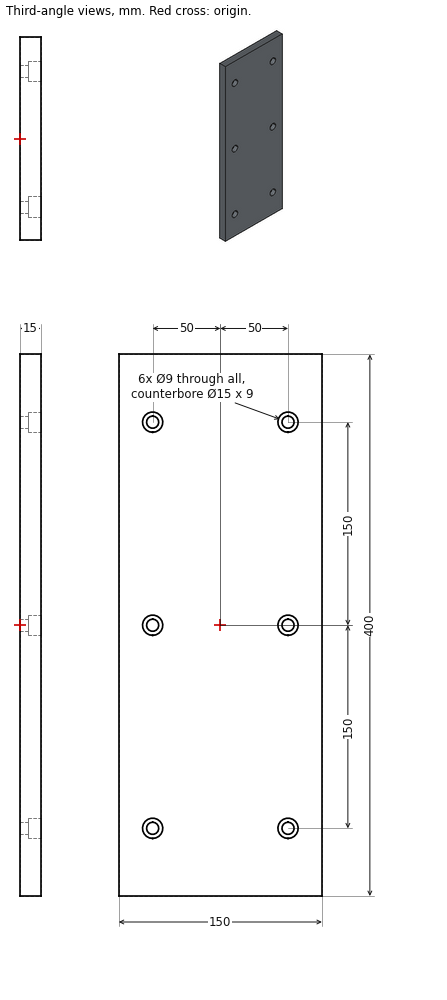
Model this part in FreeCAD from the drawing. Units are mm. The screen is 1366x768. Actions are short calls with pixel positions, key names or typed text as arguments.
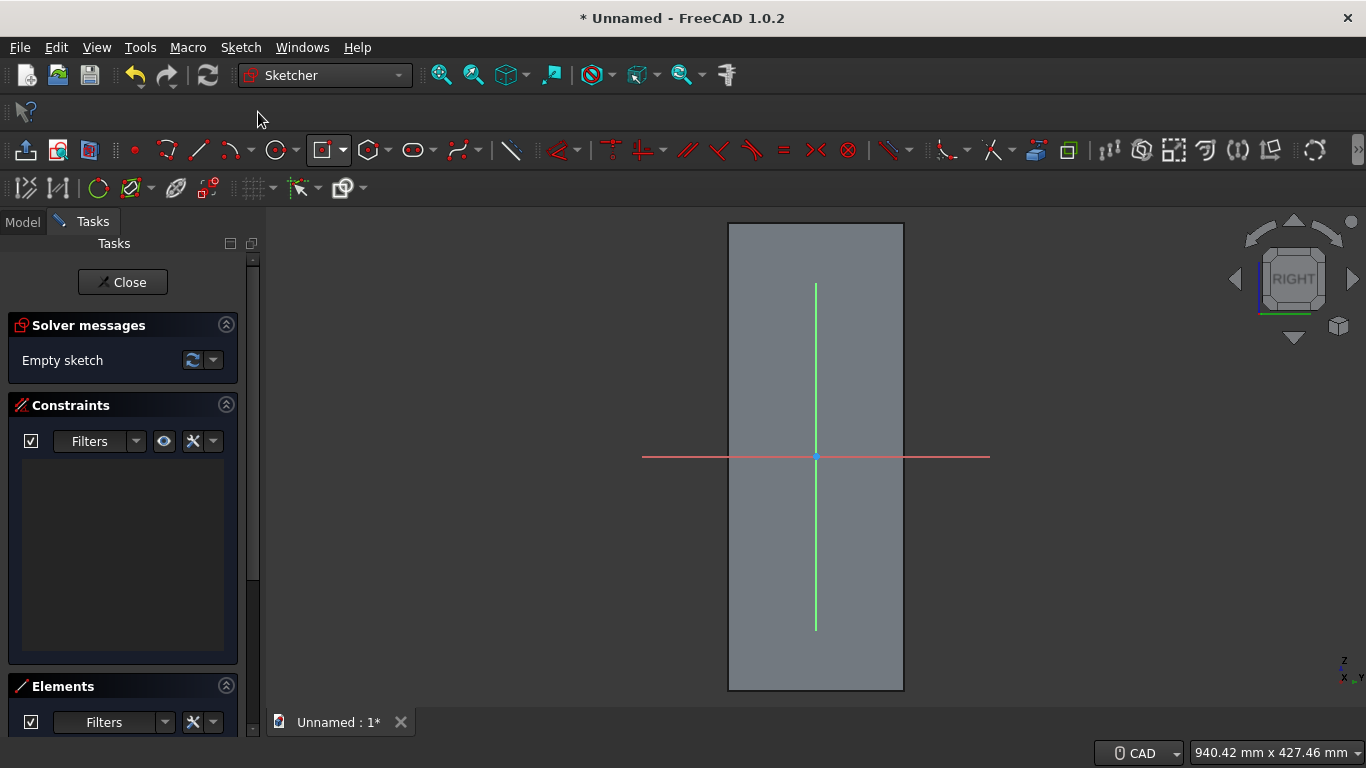
click(276, 150)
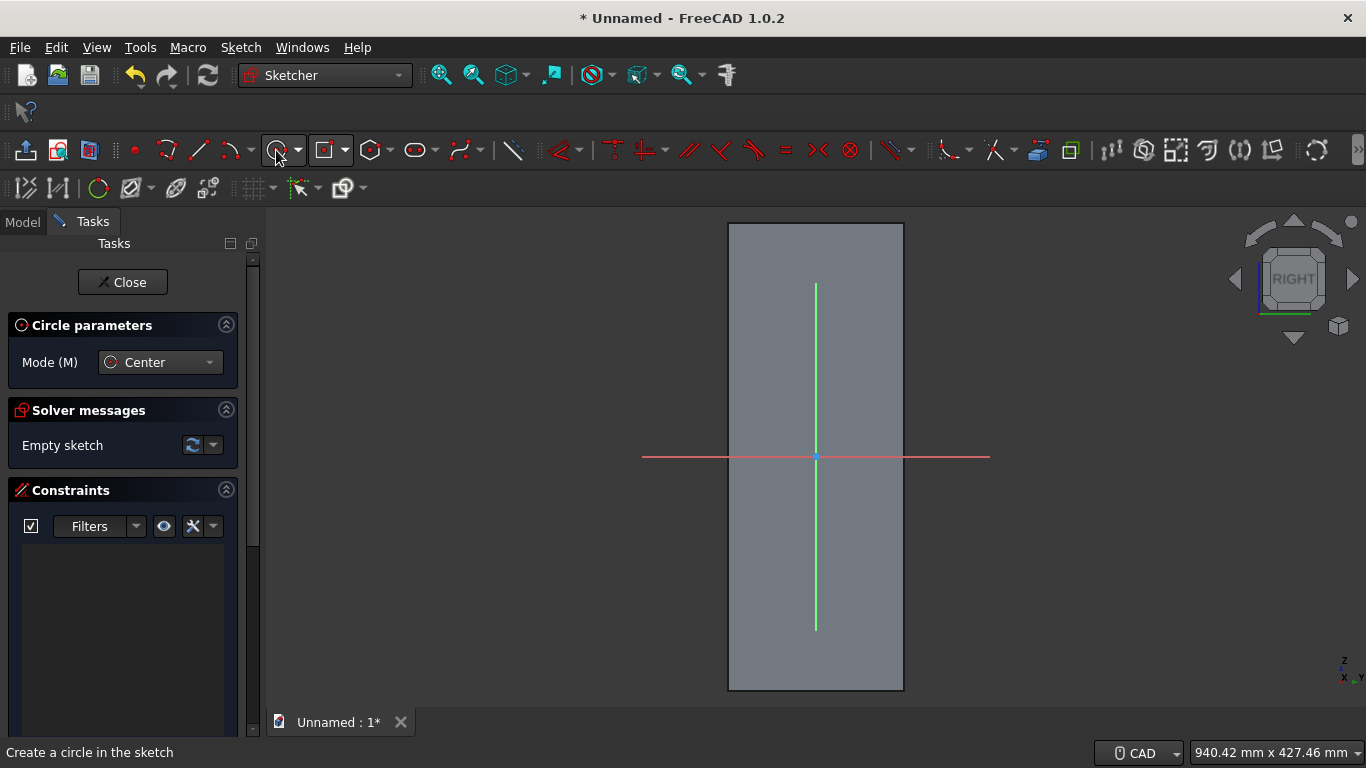
scroll(874, 282, up, 8)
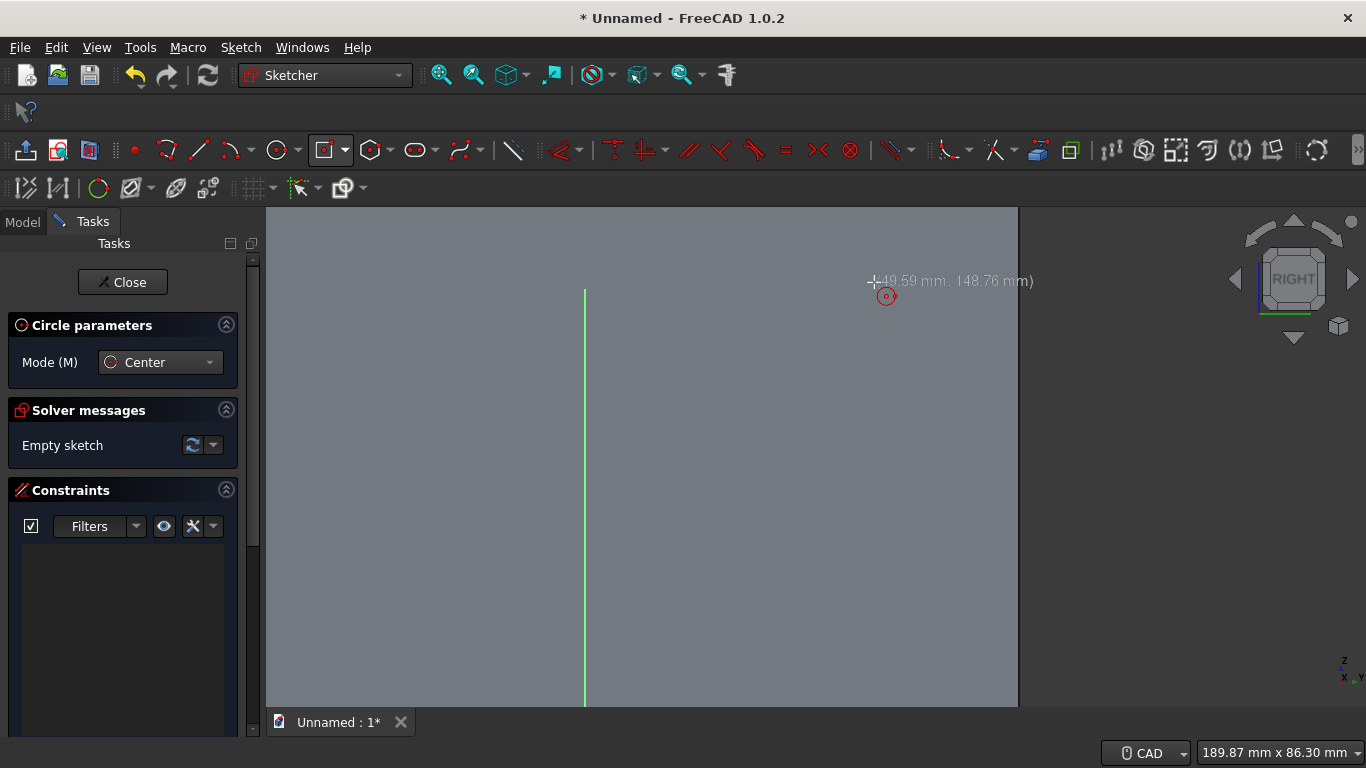
scroll(780, 320, down, 9)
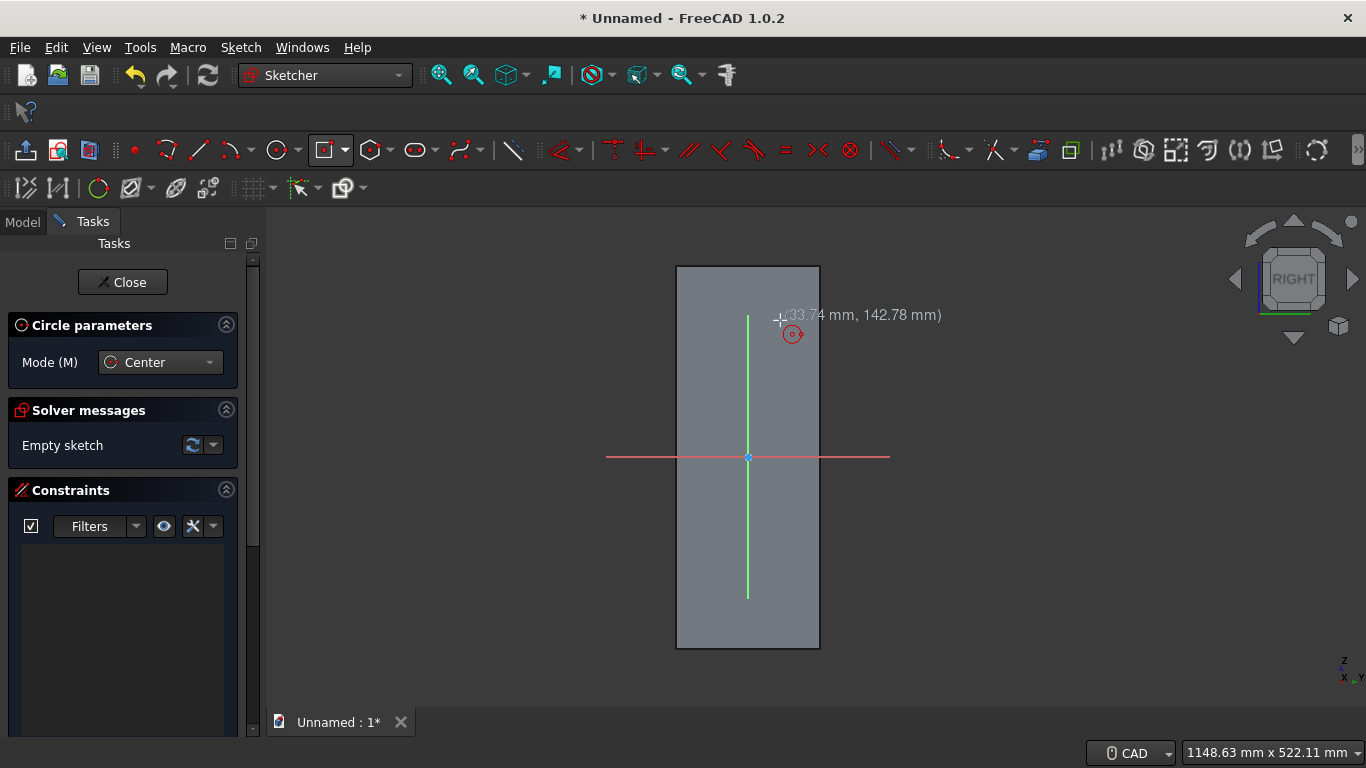
click(796, 313)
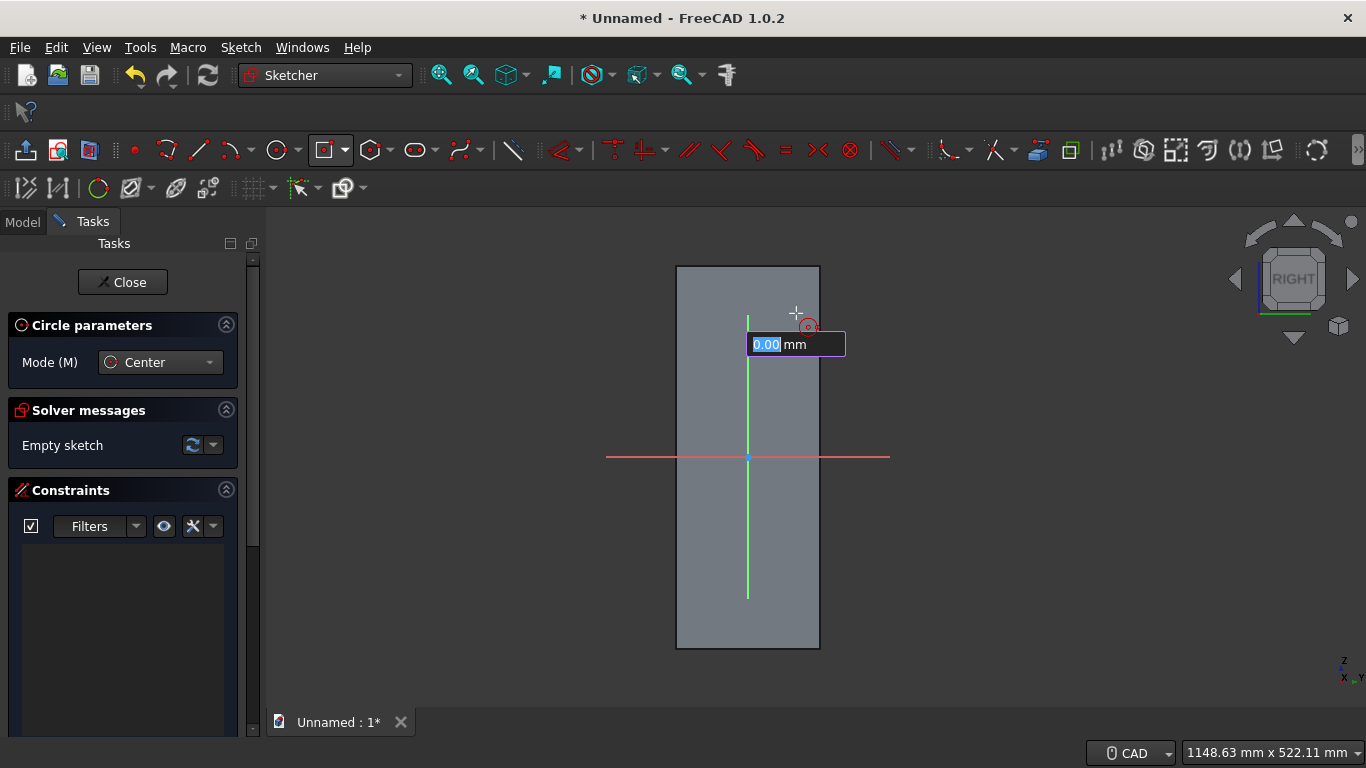
scroll(799, 310, up, 7)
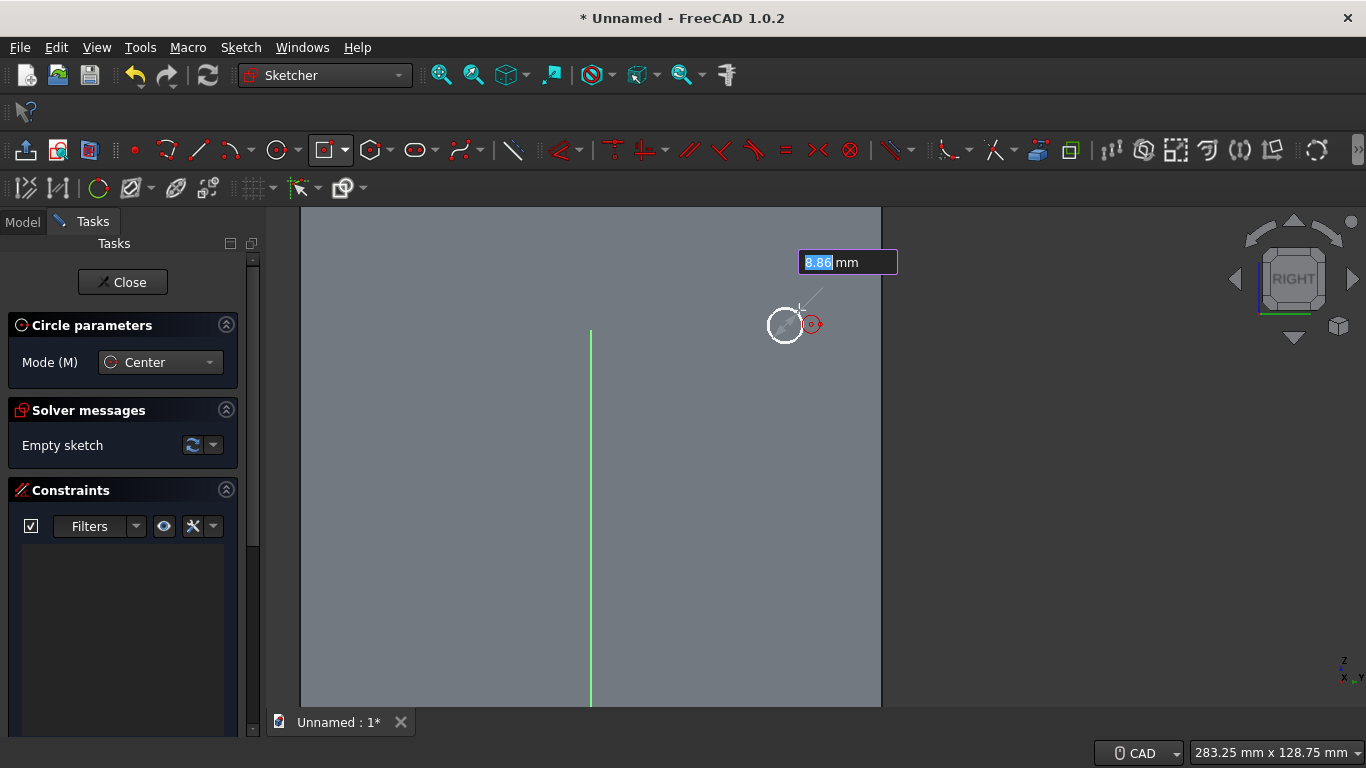
click(798, 311)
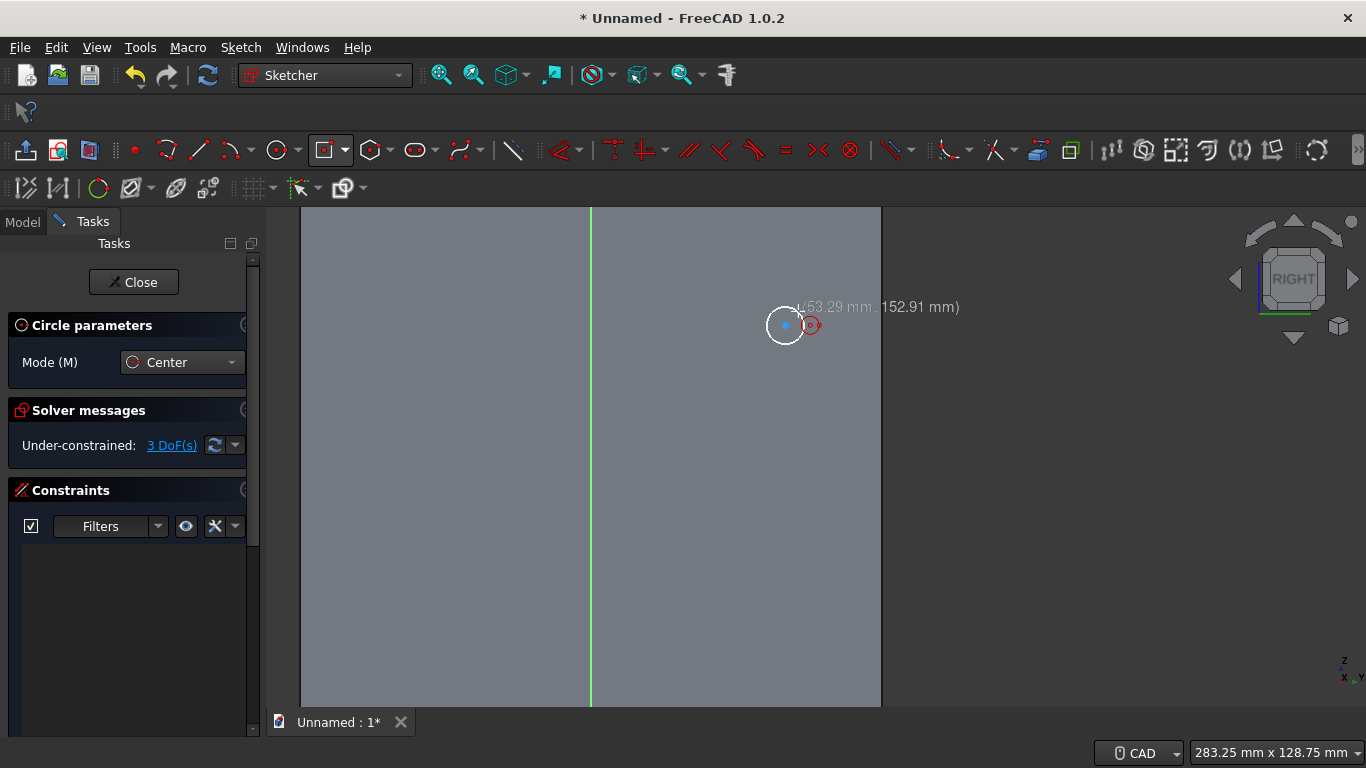
scroll(799, 310, down, 7)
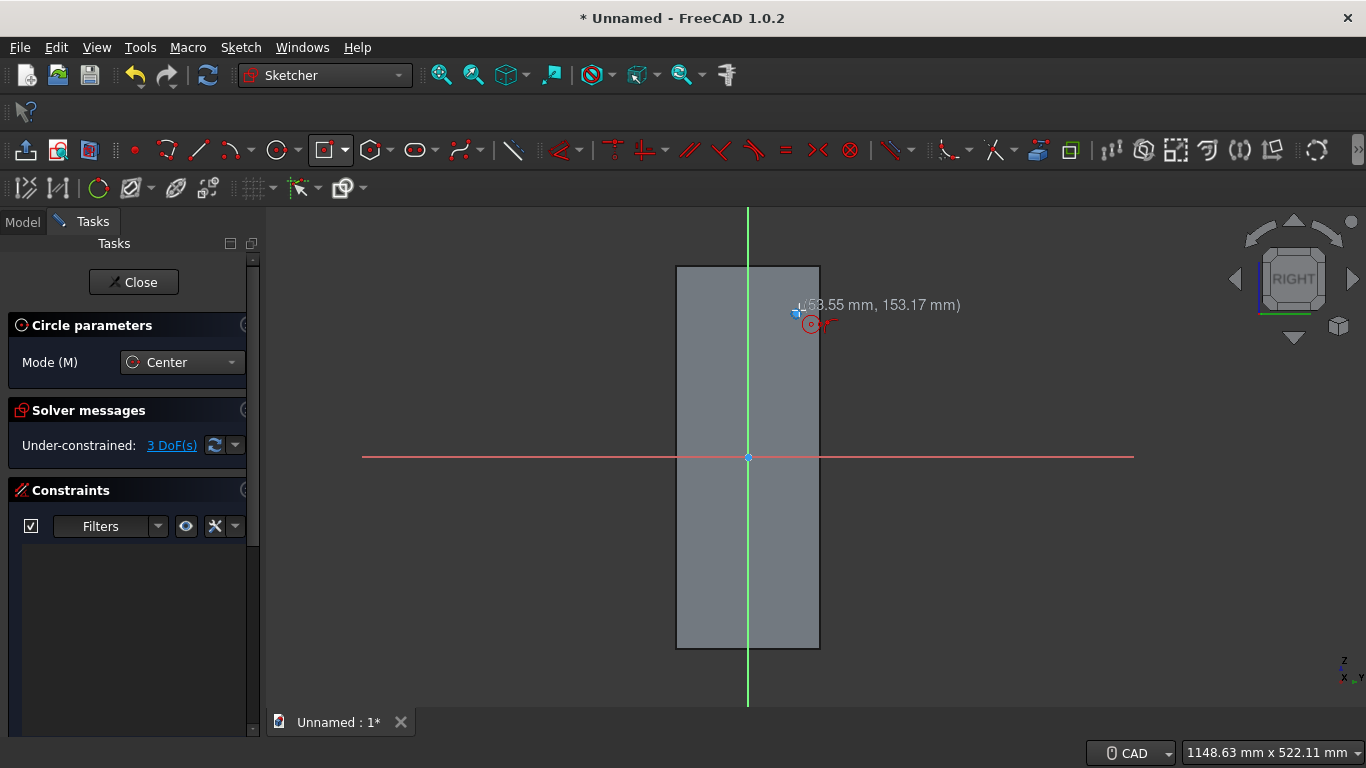
scroll(796, 457, up, 9)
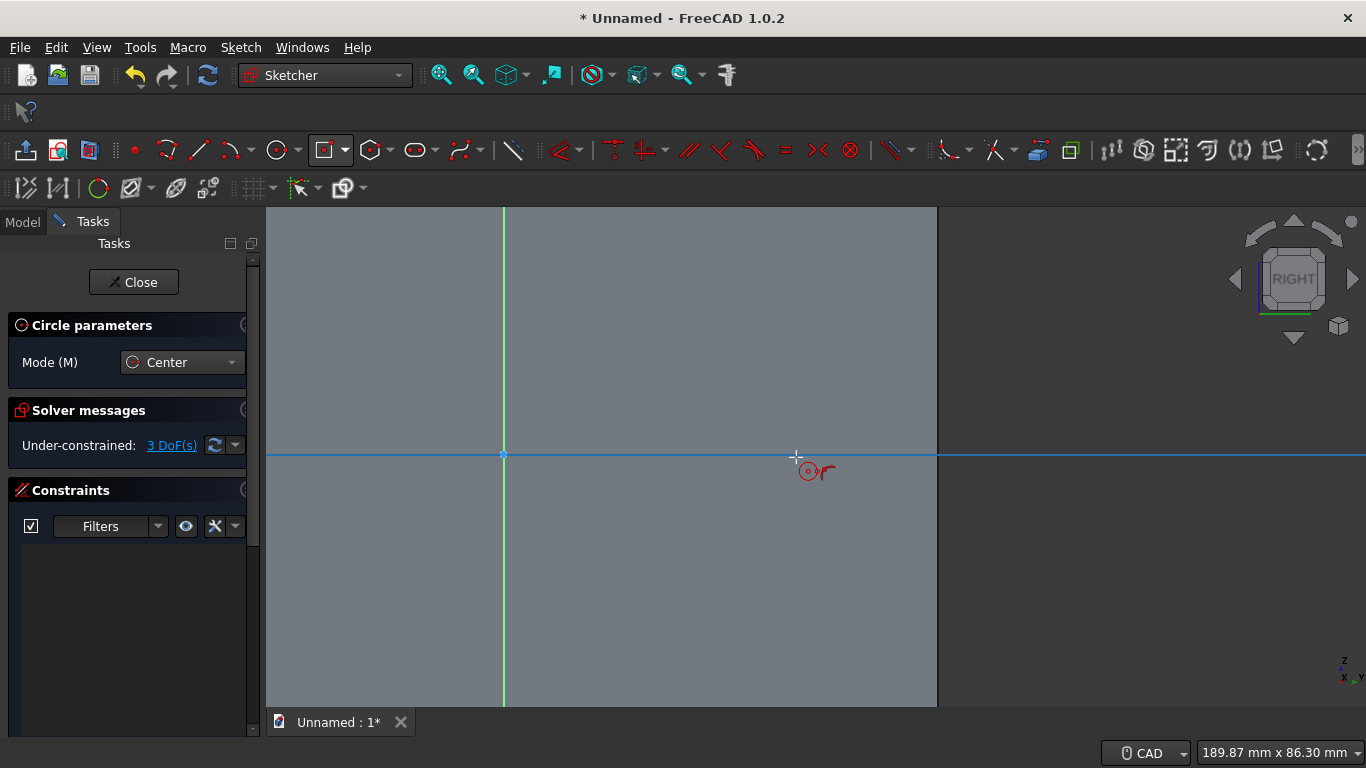
scroll(796, 457, down, 9)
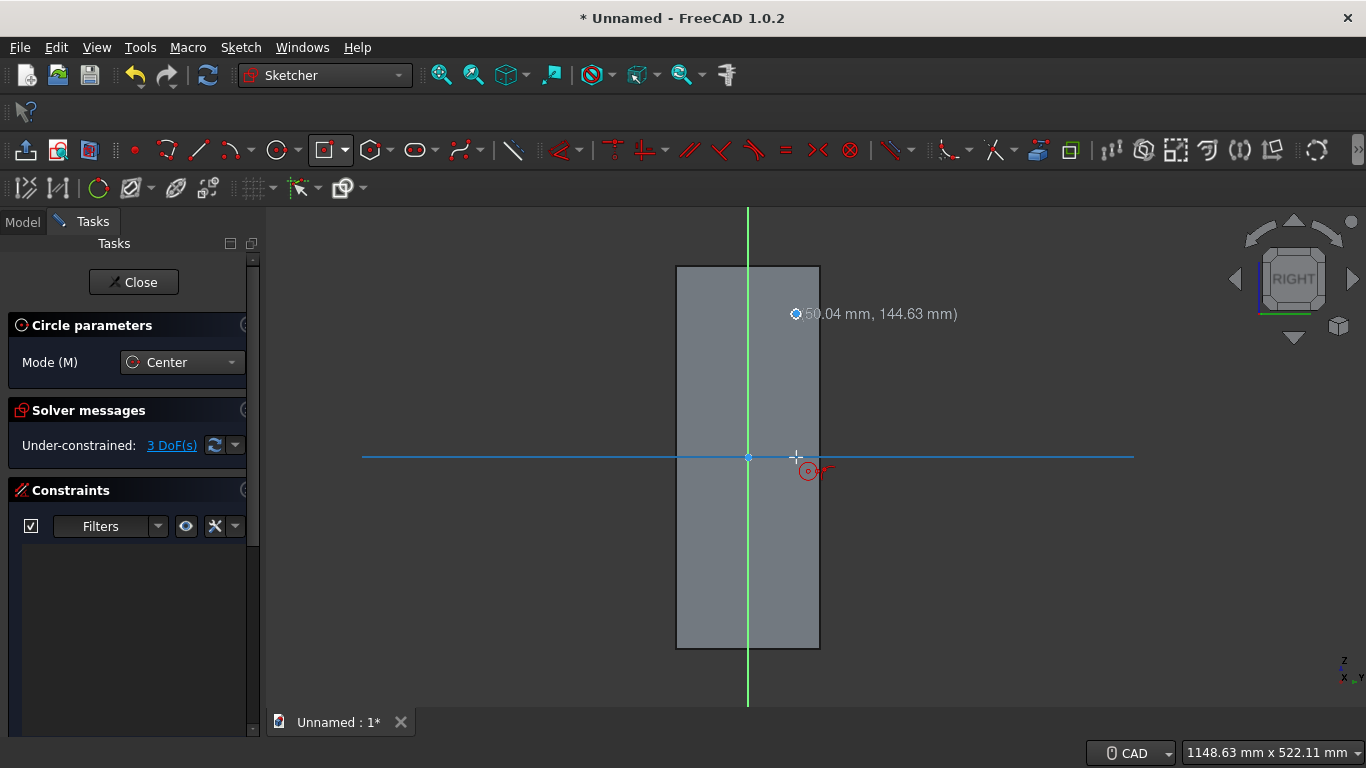
click(796, 457)